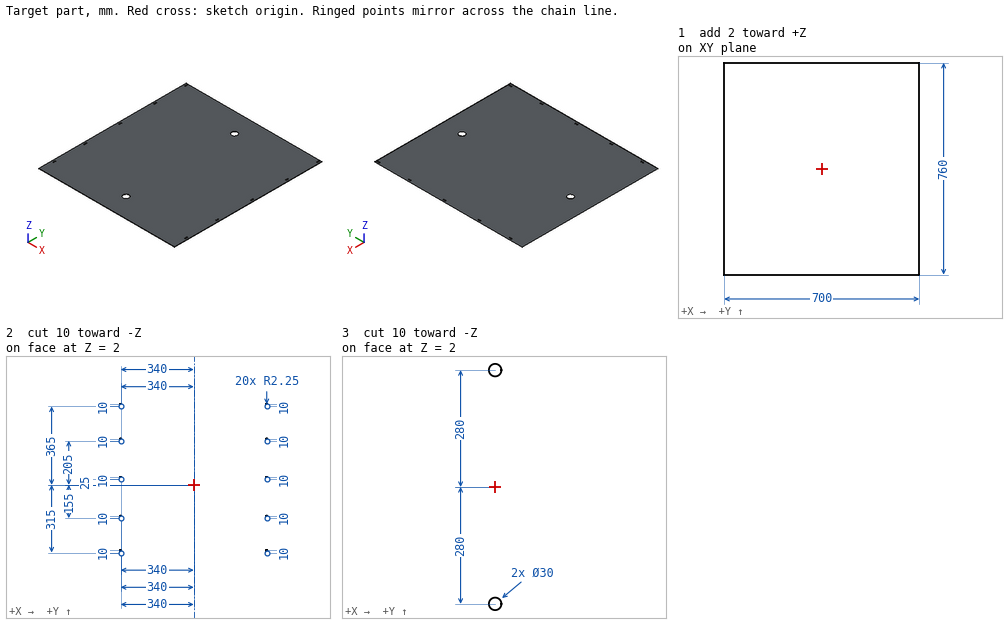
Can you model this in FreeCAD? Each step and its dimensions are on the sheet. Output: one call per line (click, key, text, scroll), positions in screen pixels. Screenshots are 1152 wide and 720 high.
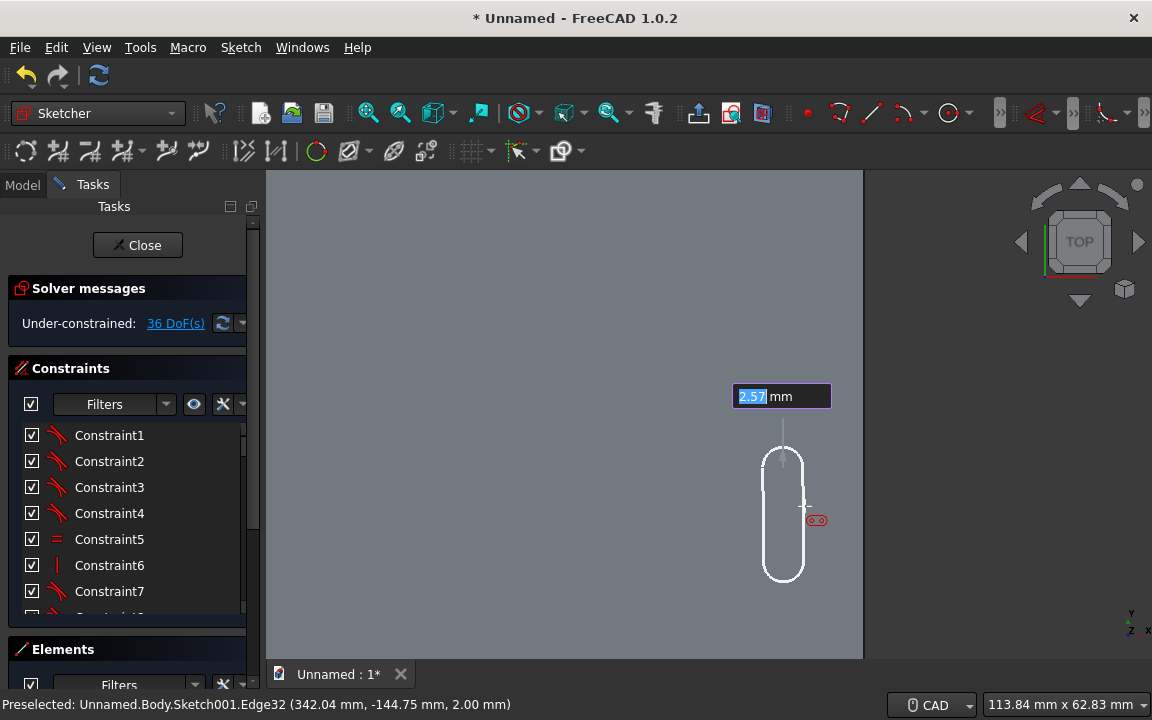
click(804, 502)
key(Escape)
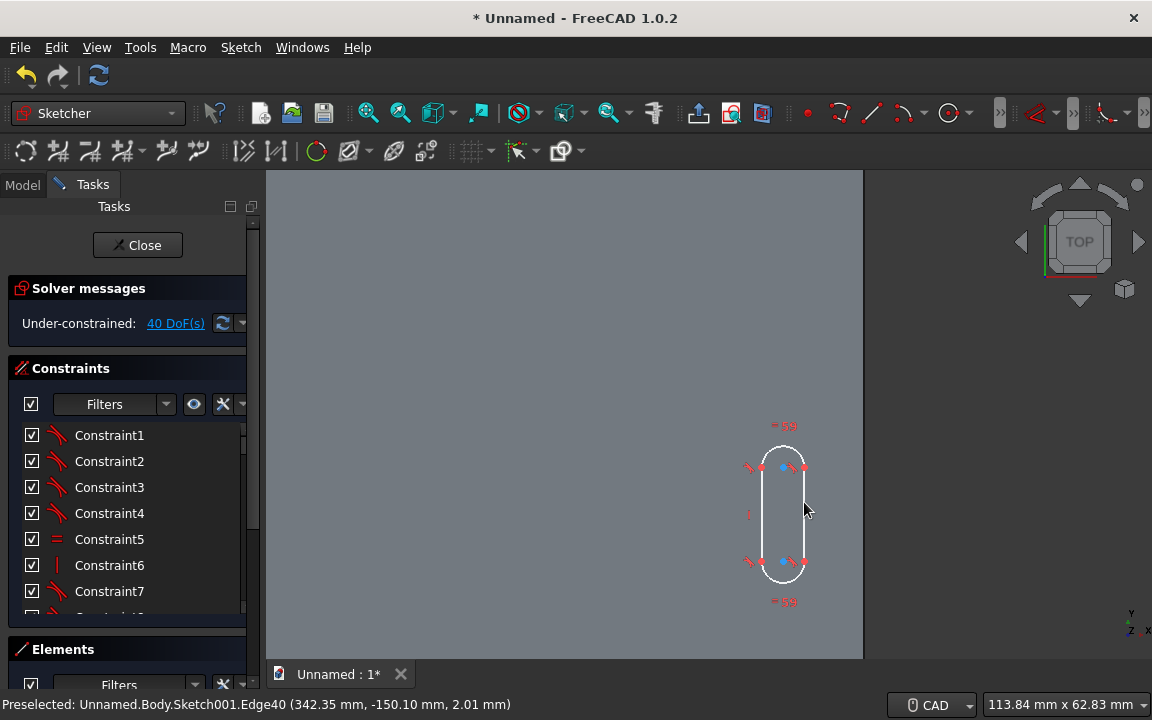
scroll(802, 500, down, 14)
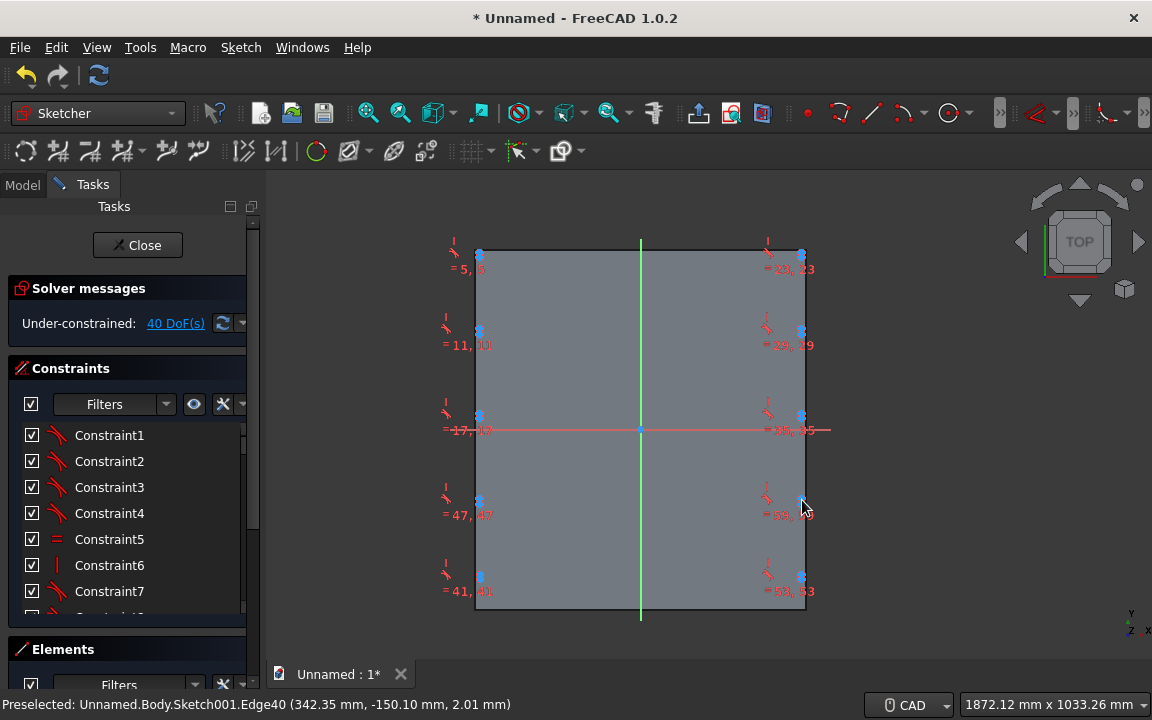
scroll(479, 259, up, 14)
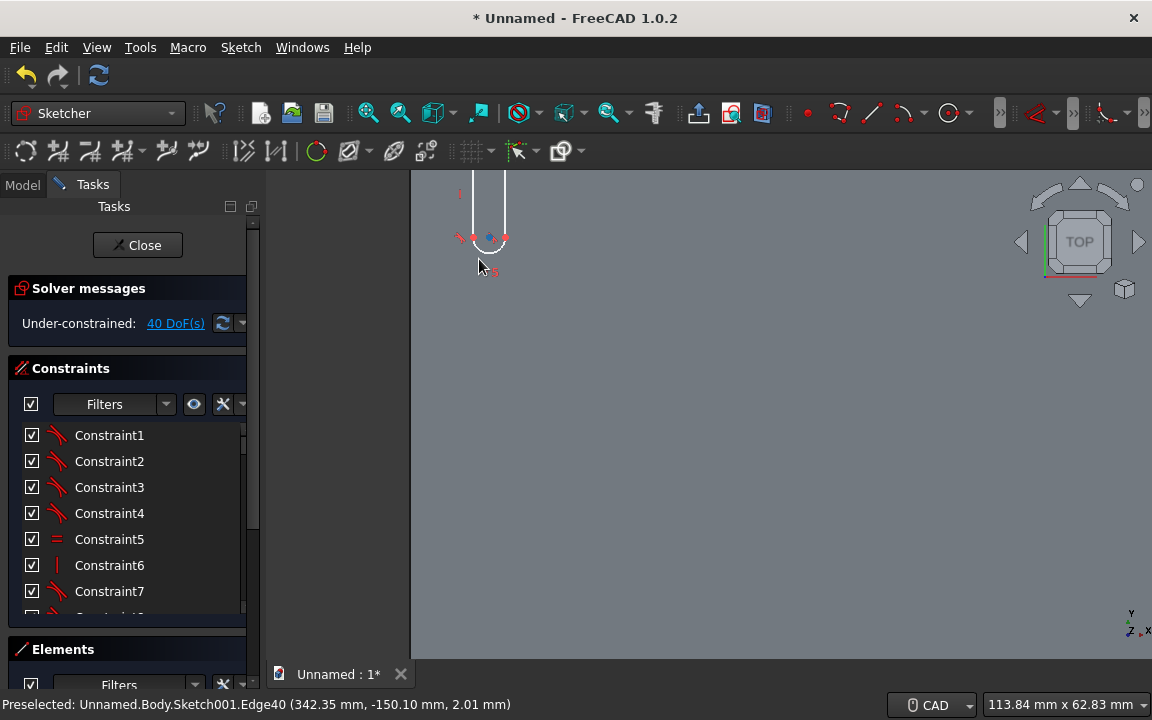
click(480, 250)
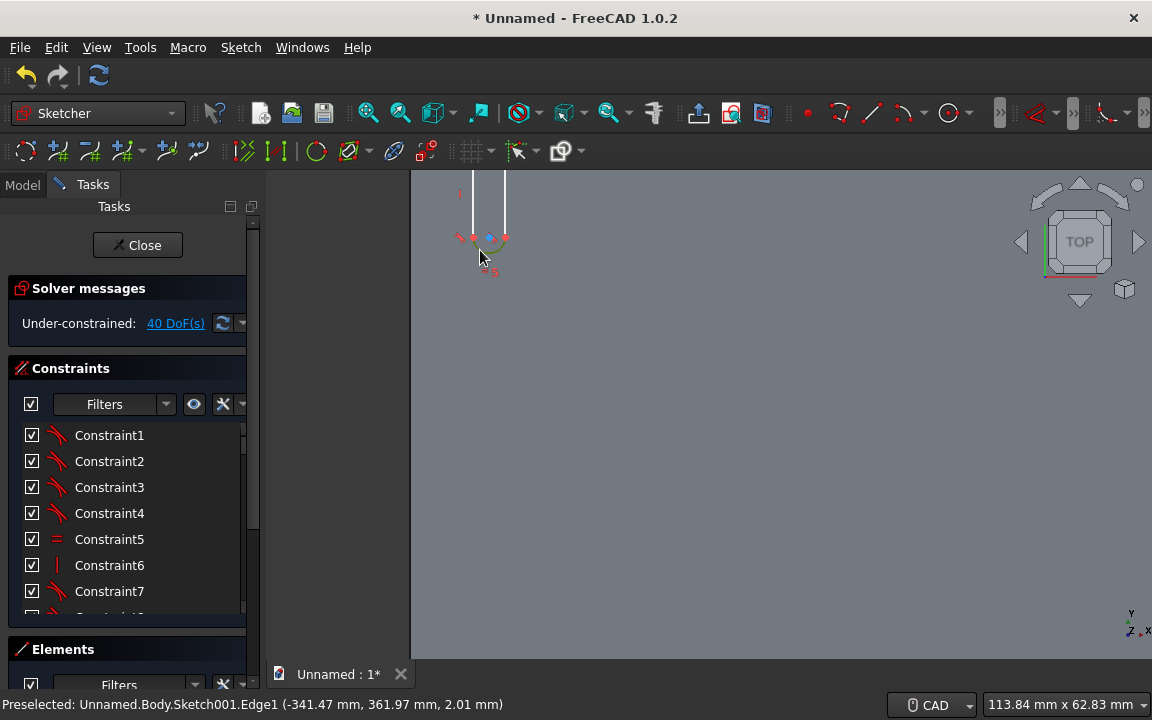
scroll(479, 258, down, 14)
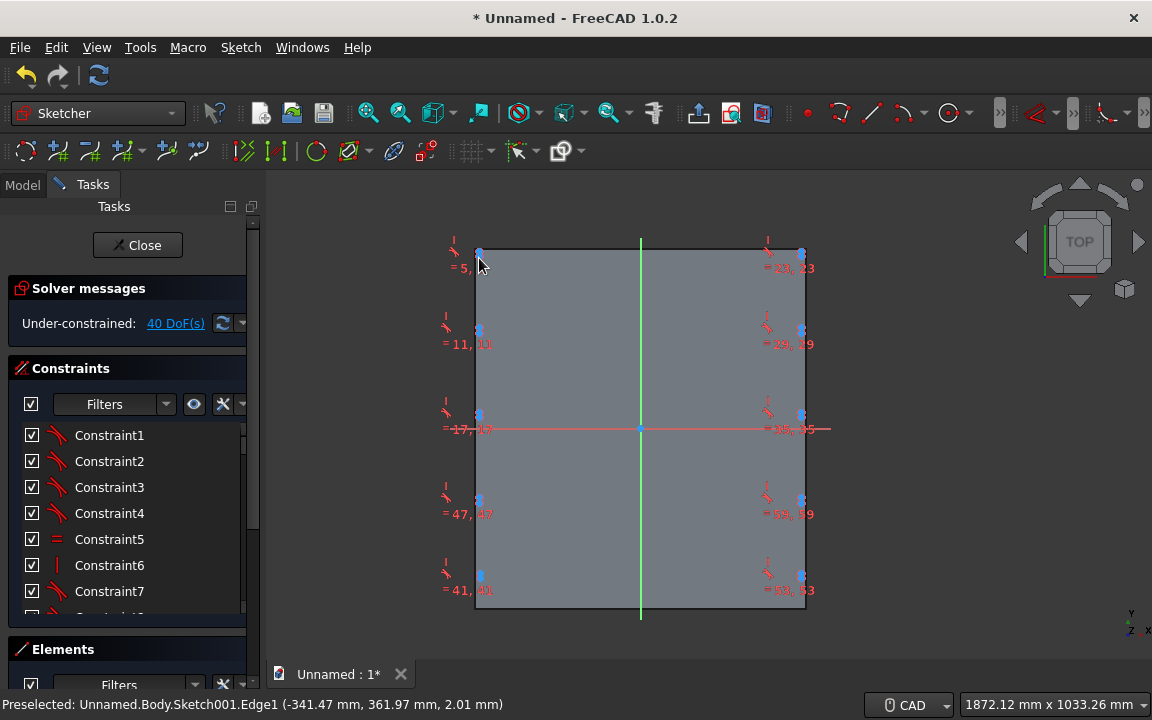
scroll(479, 334, up, 14)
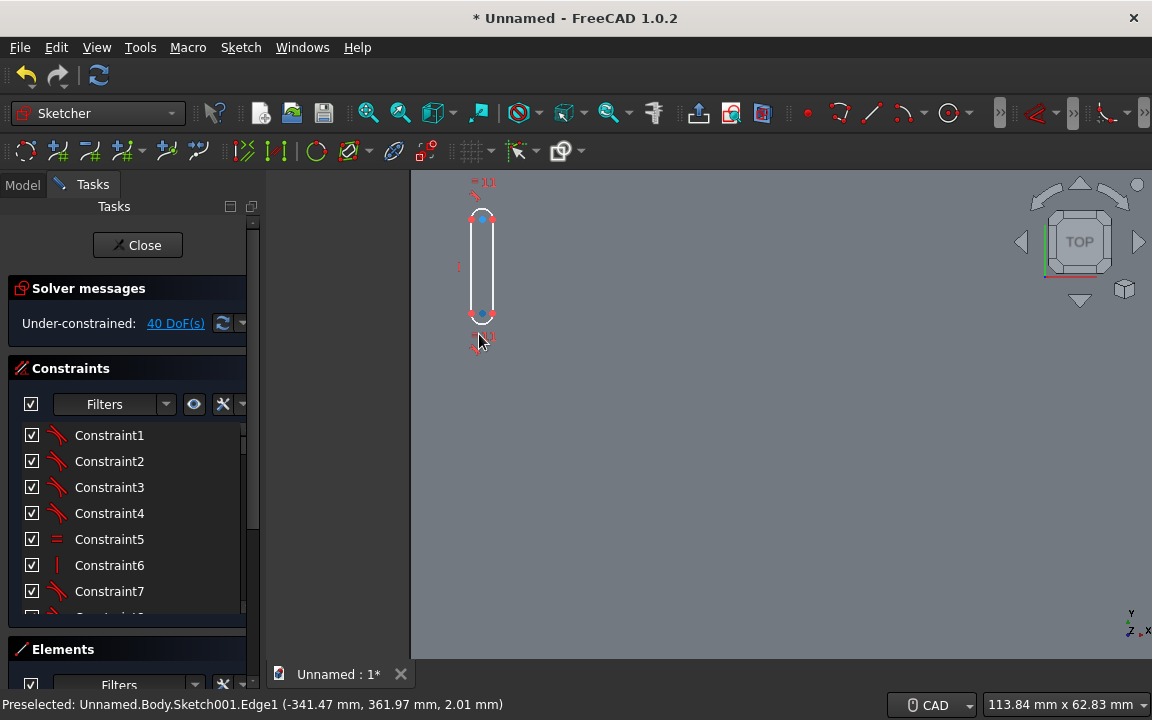
click(476, 322)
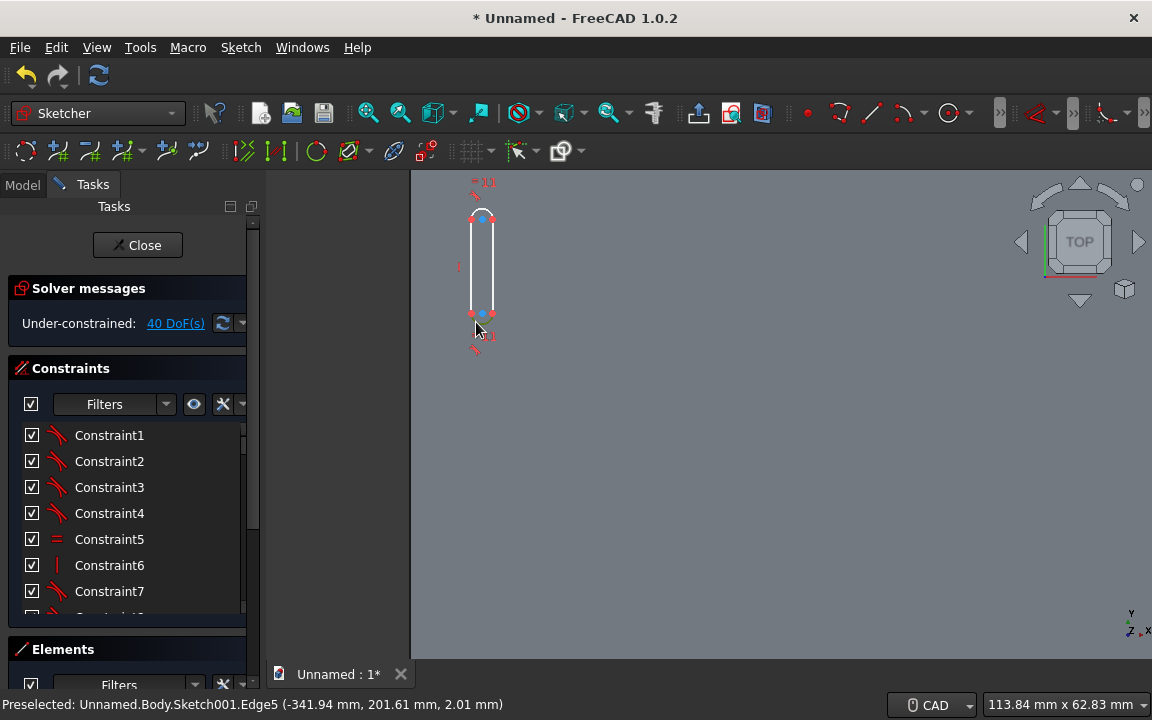
scroll(479, 334, down, 14)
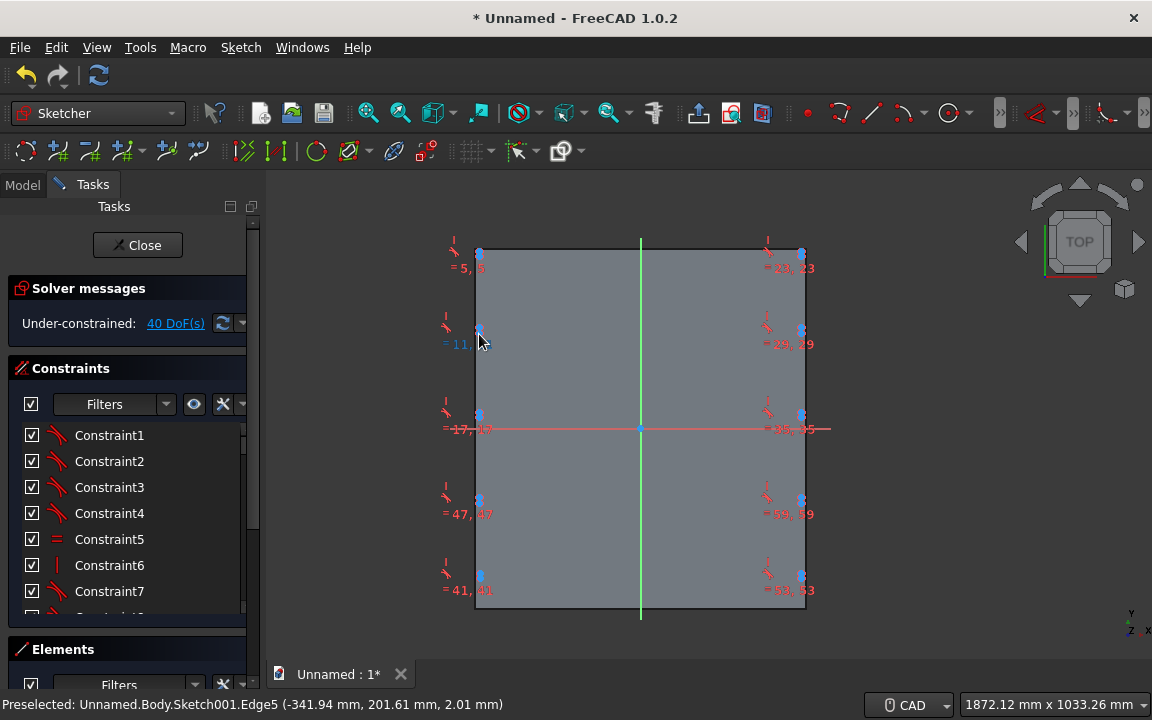
scroll(479, 419, up, 14)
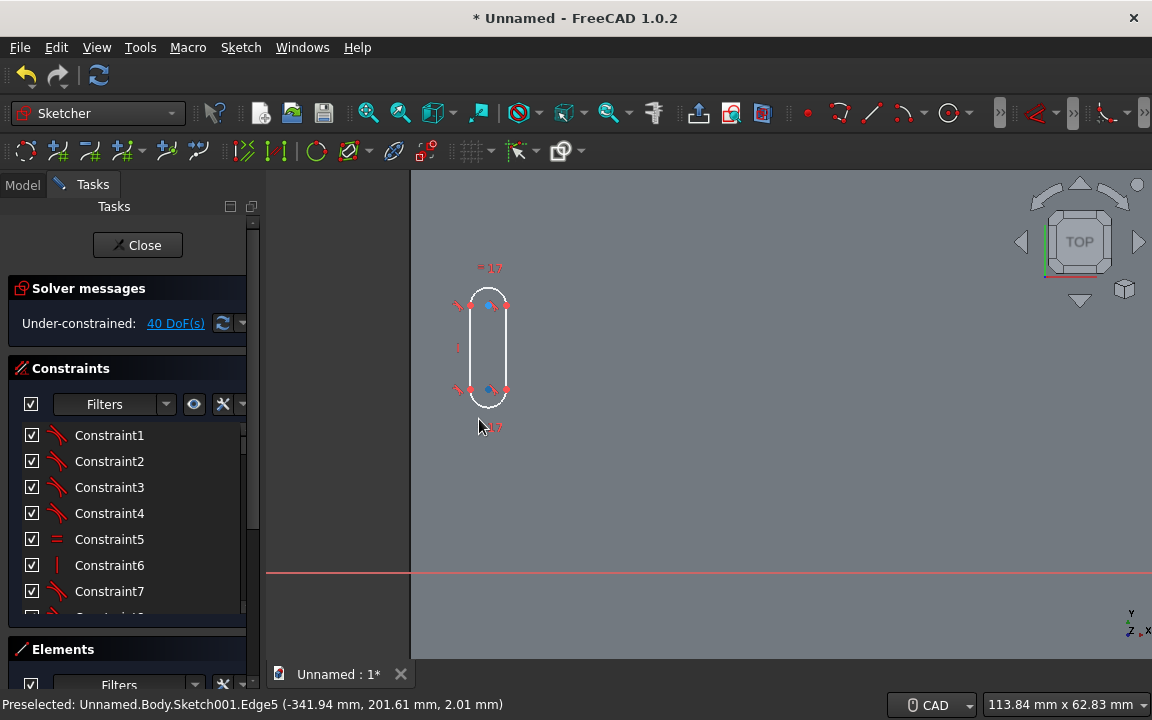
click(478, 404)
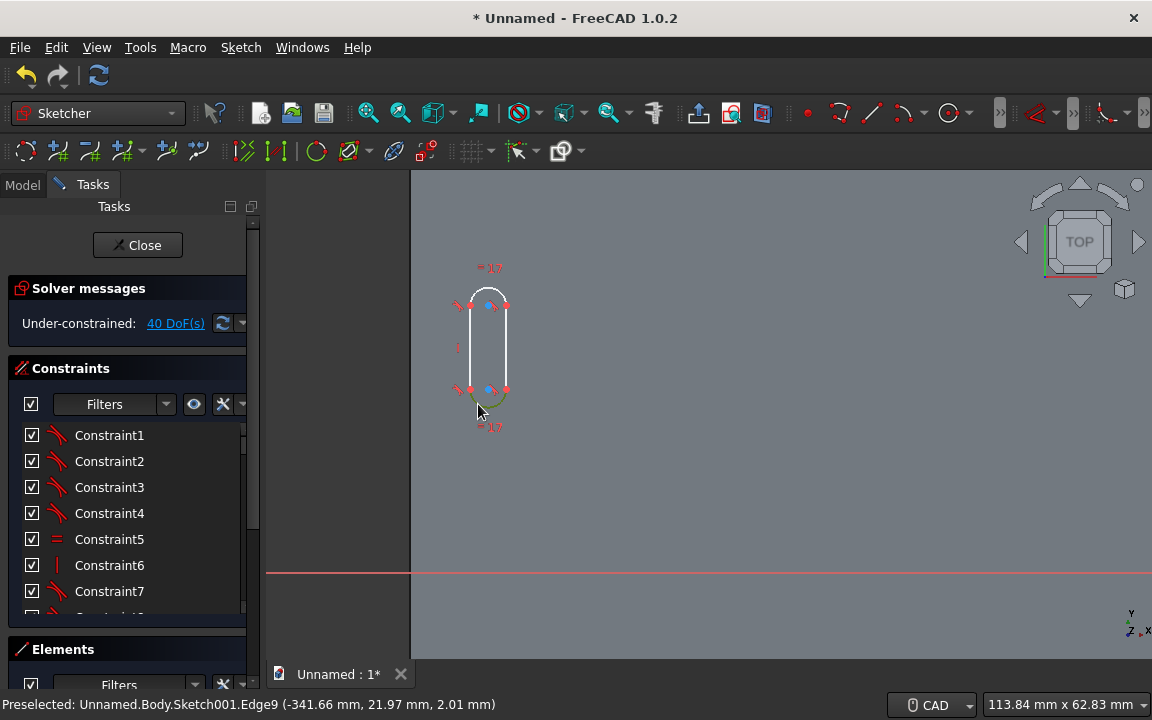
scroll(479, 419, down, 14)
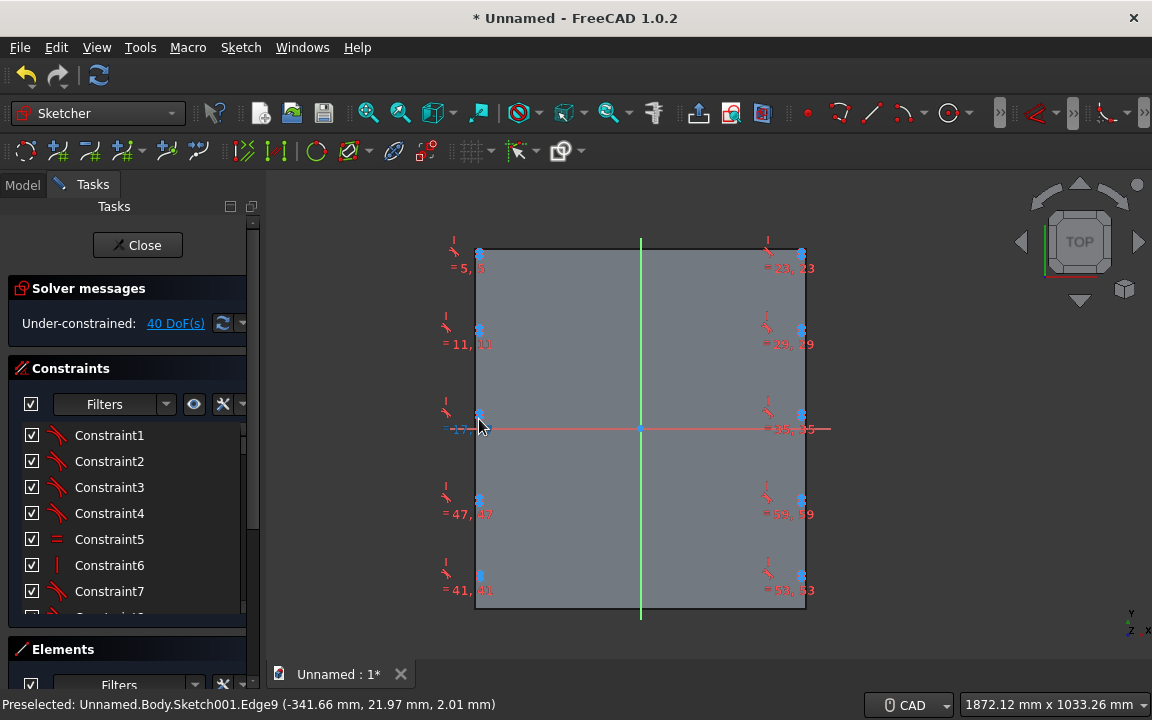
scroll(801, 258, up, 13)